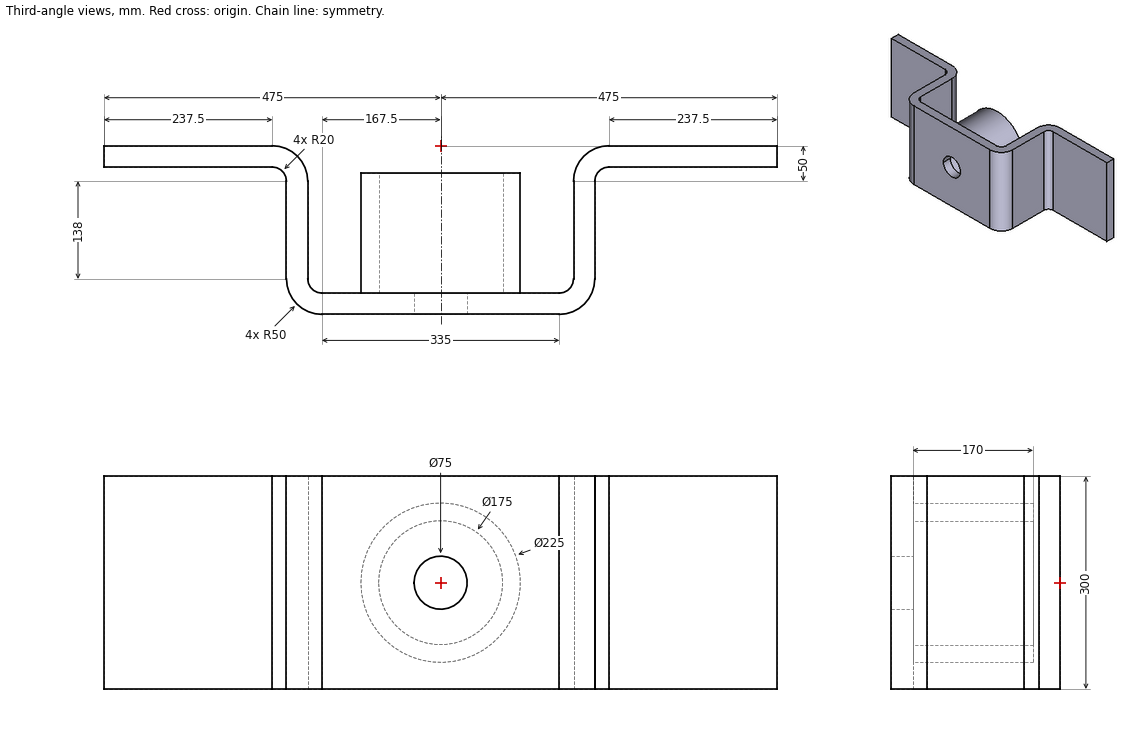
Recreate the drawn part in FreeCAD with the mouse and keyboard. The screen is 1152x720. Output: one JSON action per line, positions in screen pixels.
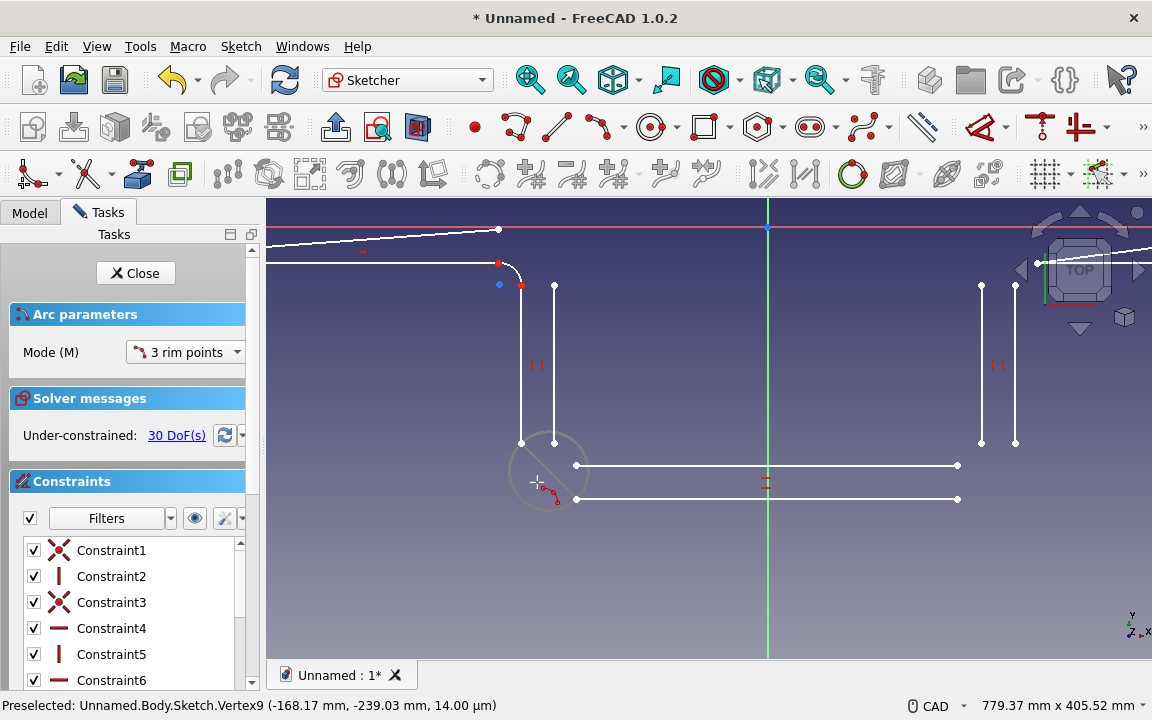
{"action": "left_click", "coordinate": [537, 481]}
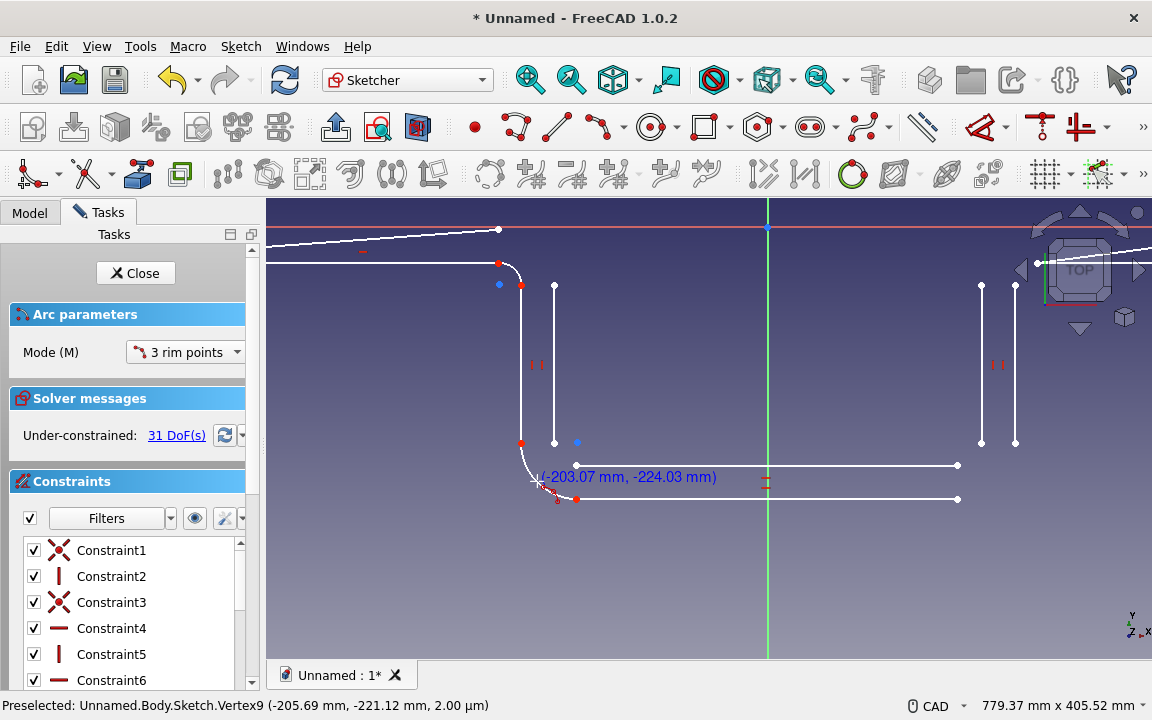
{"action": "left_click", "coordinate": [957, 499]}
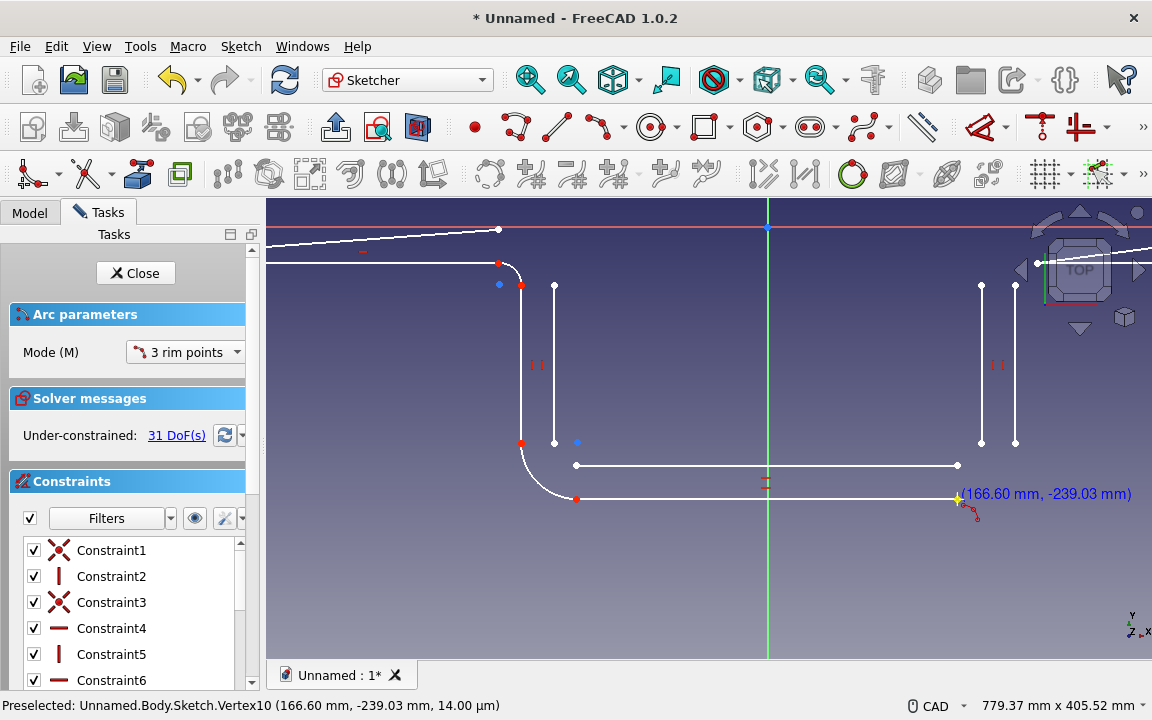
{"action": "scroll", "coordinate": [537, 482], "scroll_direction": "down", "scroll_amount": 4}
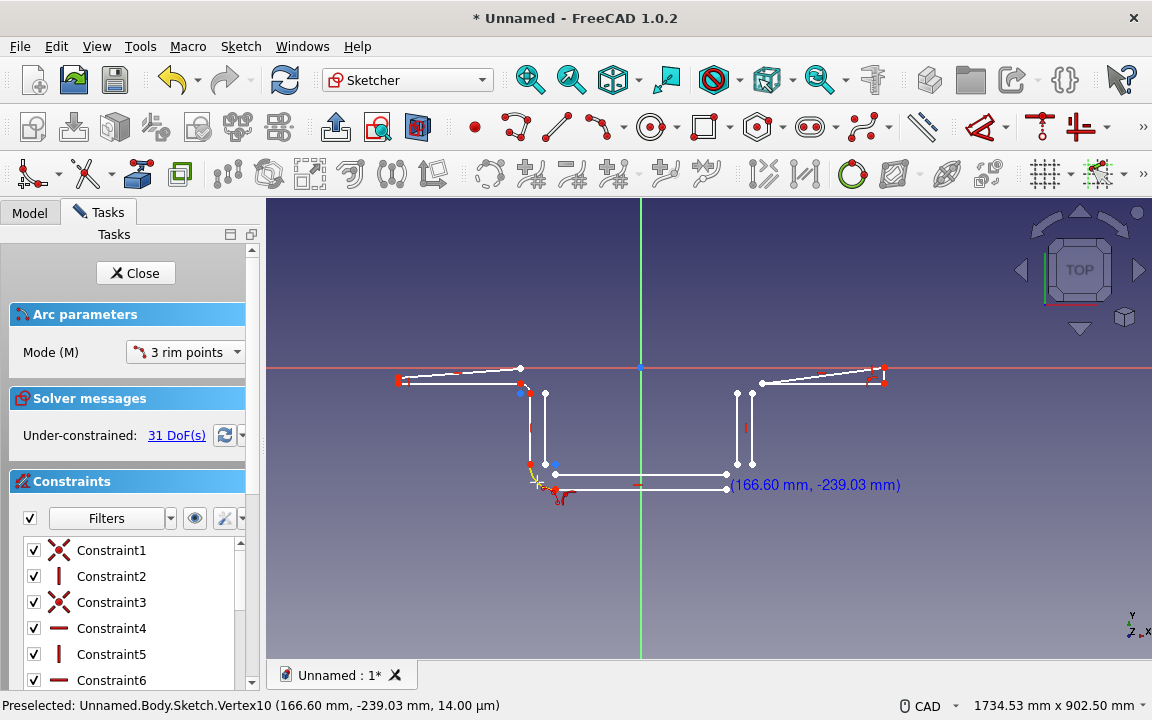
{"action": "left_click", "coordinate": [752, 465]}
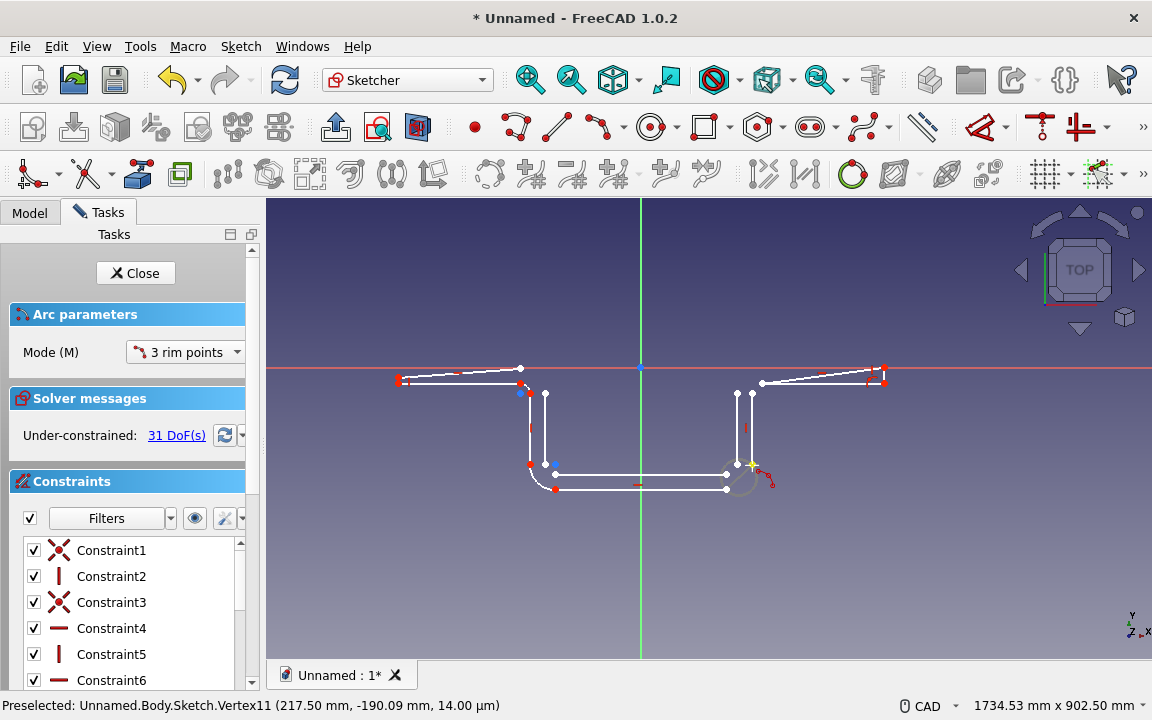
{"action": "scroll", "coordinate": [745, 482], "scroll_direction": "up", "scroll_amount": 4}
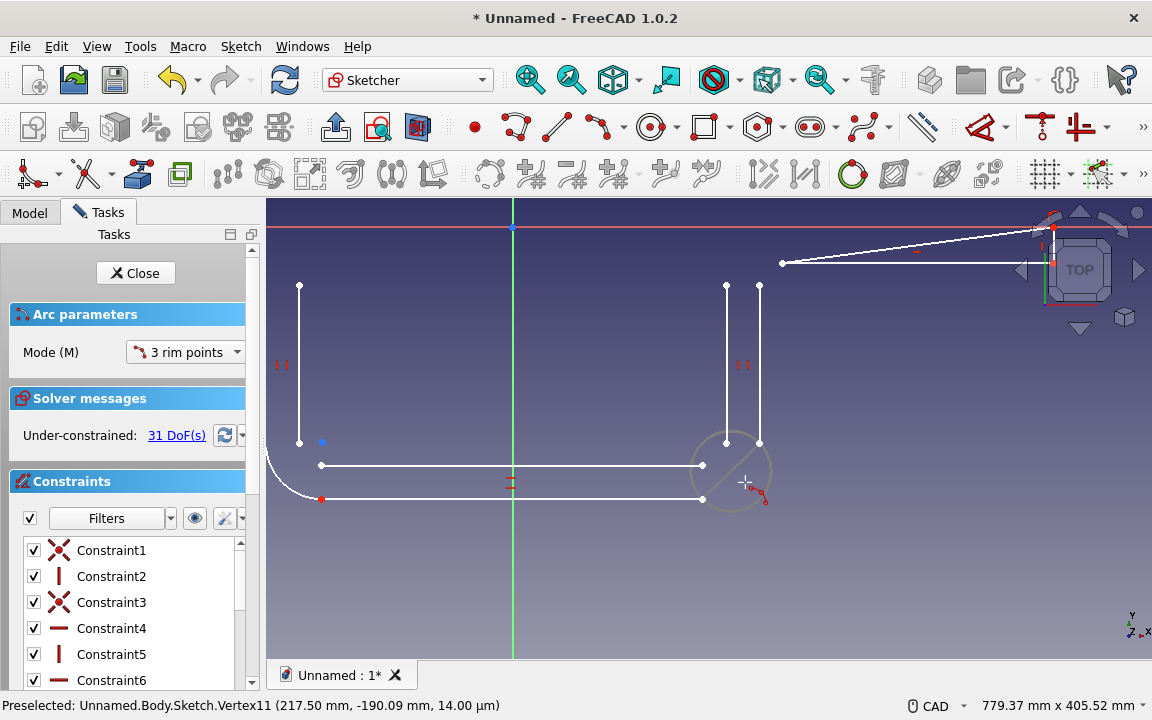
{"action": "left_click", "coordinate": [743, 481]}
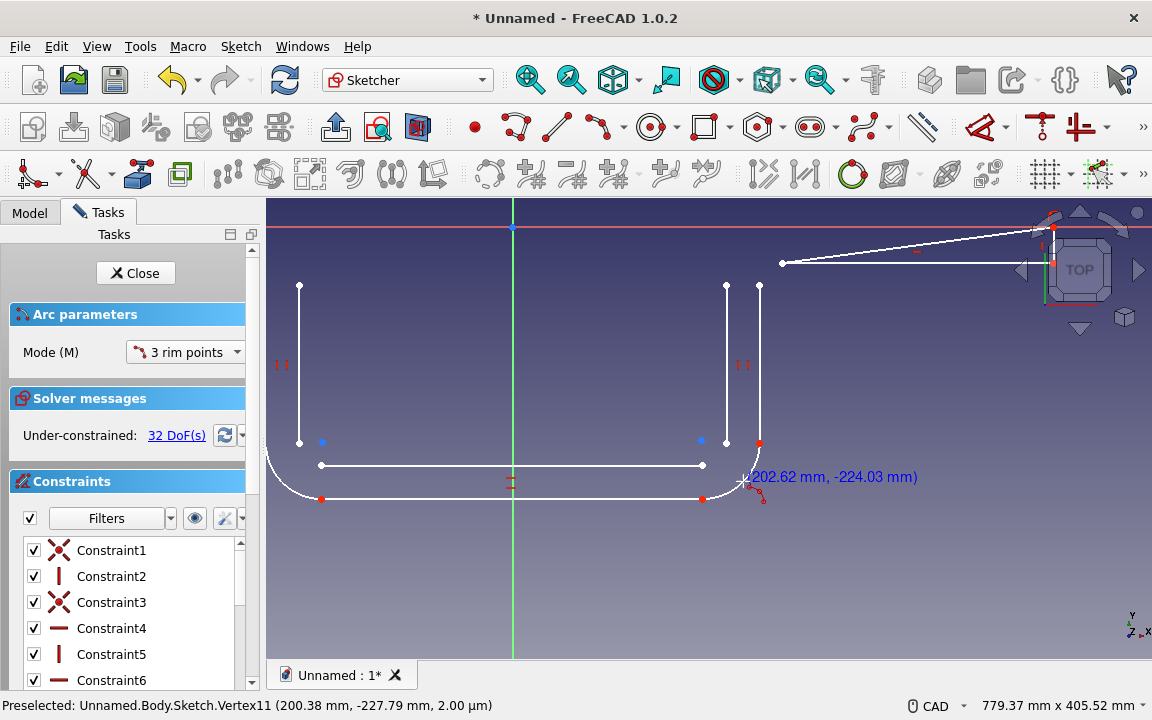
{"action": "left_click", "coordinate": [760, 285]}
{"action": "left_click", "coordinate": [782, 263]}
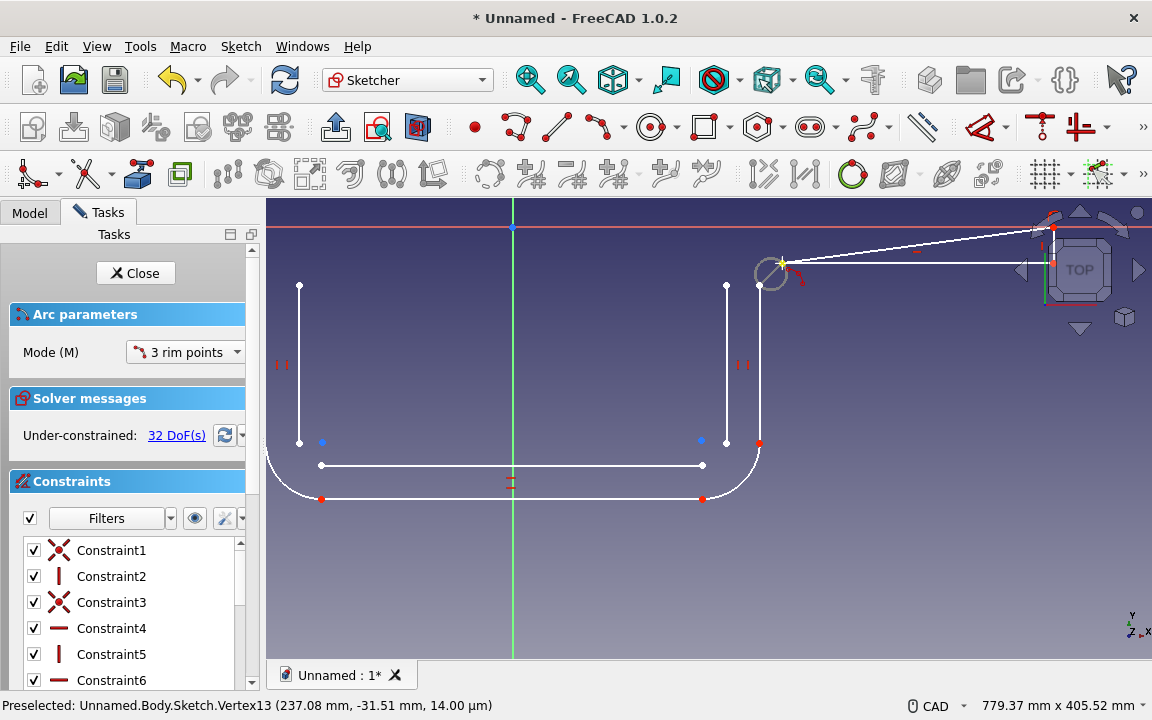
{"action": "scroll", "coordinate": [767, 268], "scroll_direction": "up", "scroll_amount": 5}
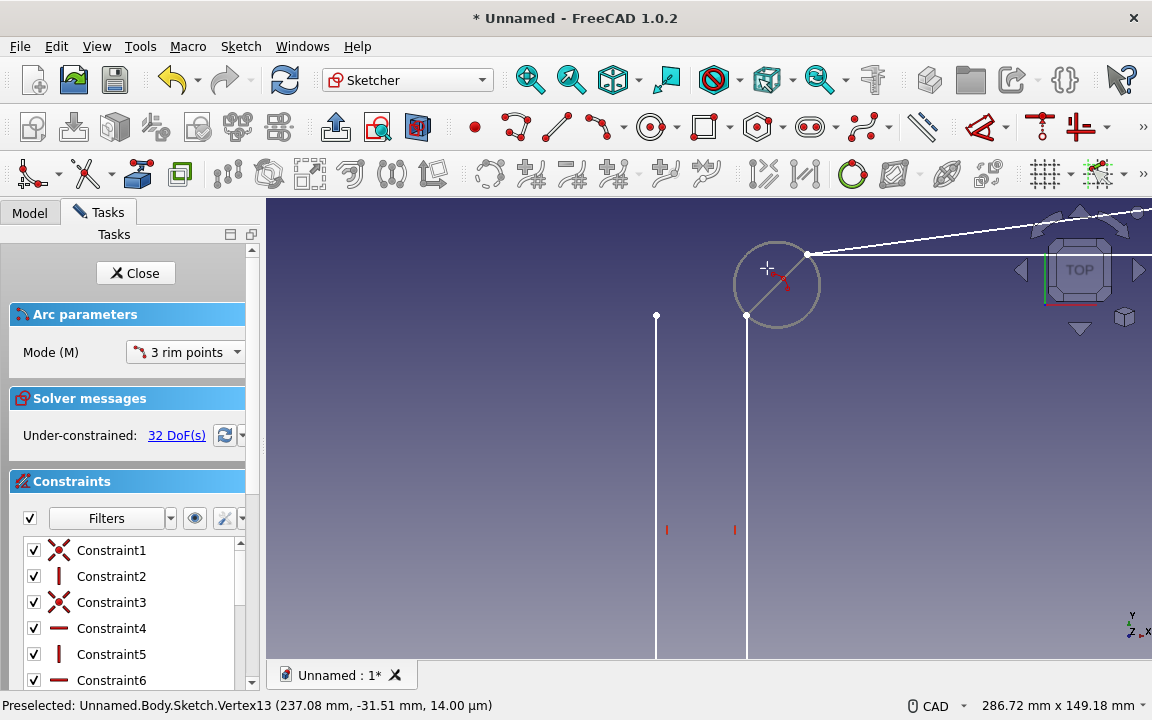
{"action": "left_click", "coordinate": [765, 268]}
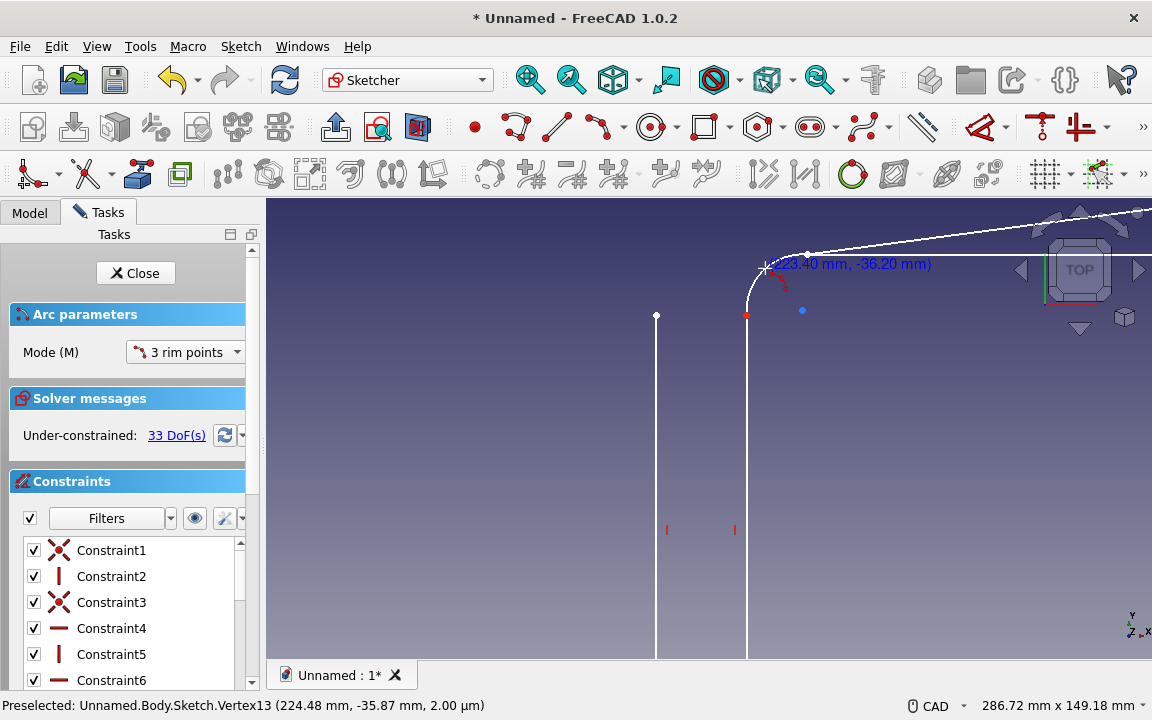
{"action": "scroll", "coordinate": [753, 409], "scroll_direction": "down", "scroll_amount": 9}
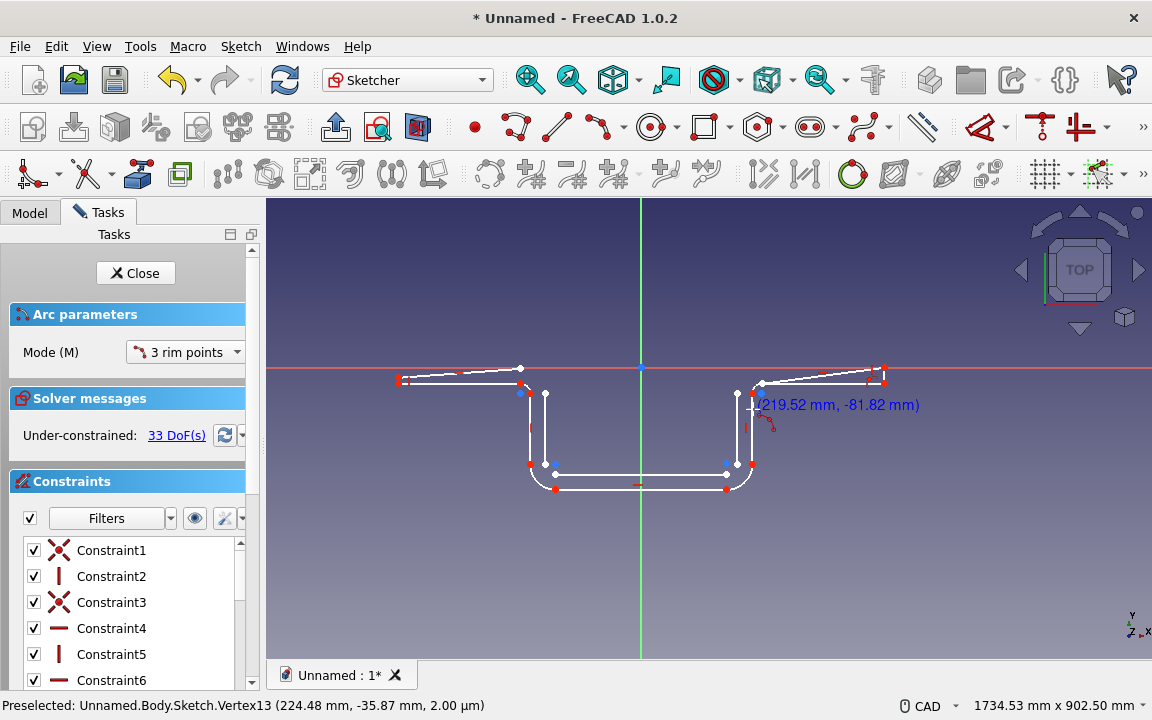
{"action": "left_click", "coordinate": [762, 384]}
{"action": "left_click", "coordinate": [737, 394]}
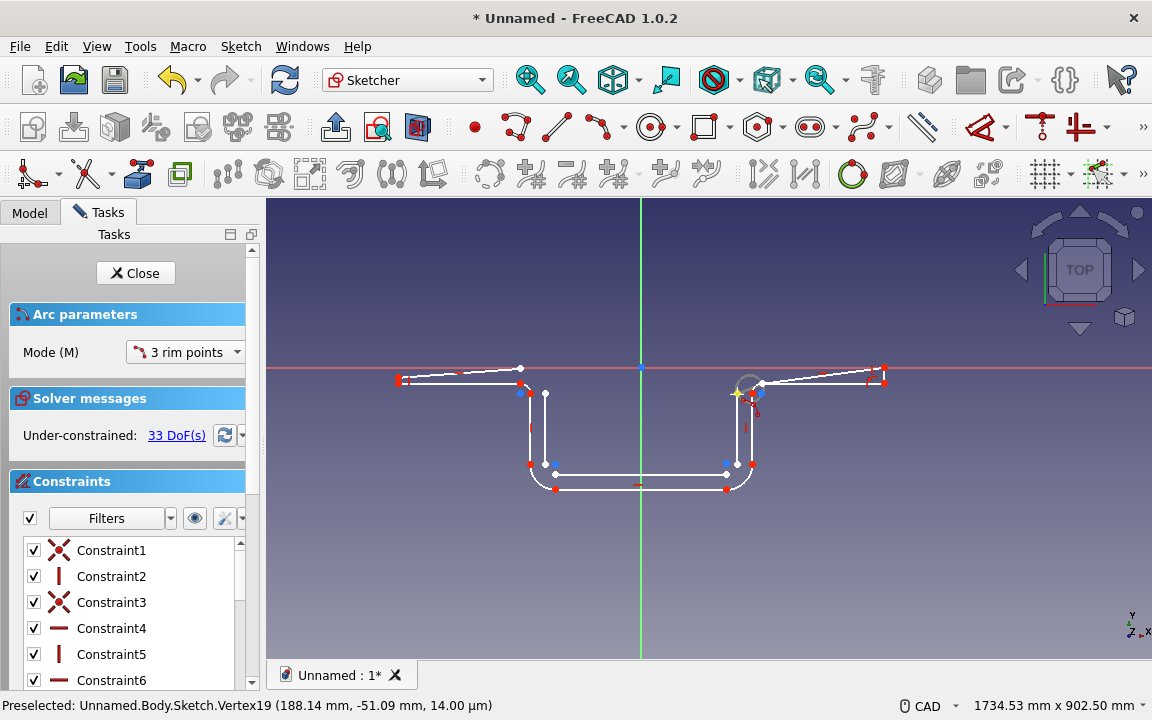
{"action": "scroll", "coordinate": [745, 375], "scroll_direction": "up", "scroll_amount": 4}